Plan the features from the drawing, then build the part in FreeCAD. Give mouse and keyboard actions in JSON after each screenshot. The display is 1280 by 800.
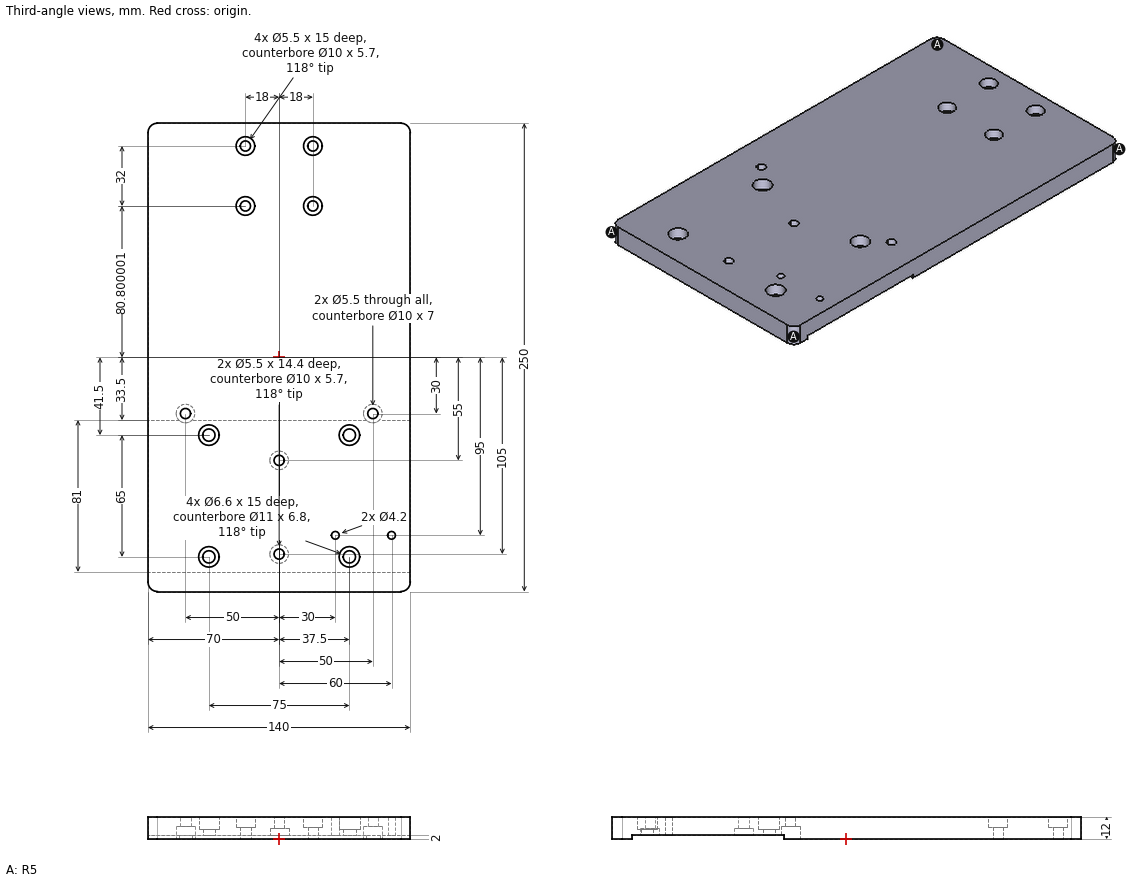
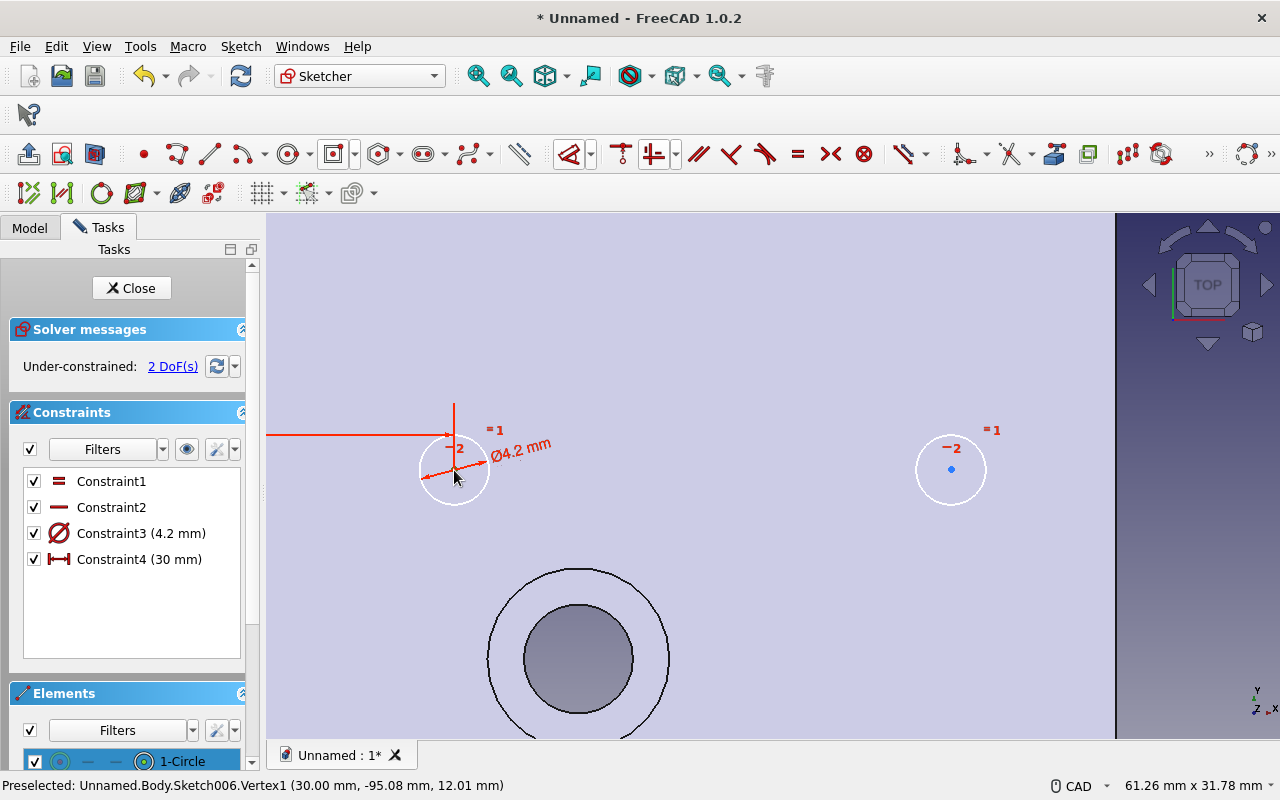
{"action": "left_click", "coordinate": [590, 154]}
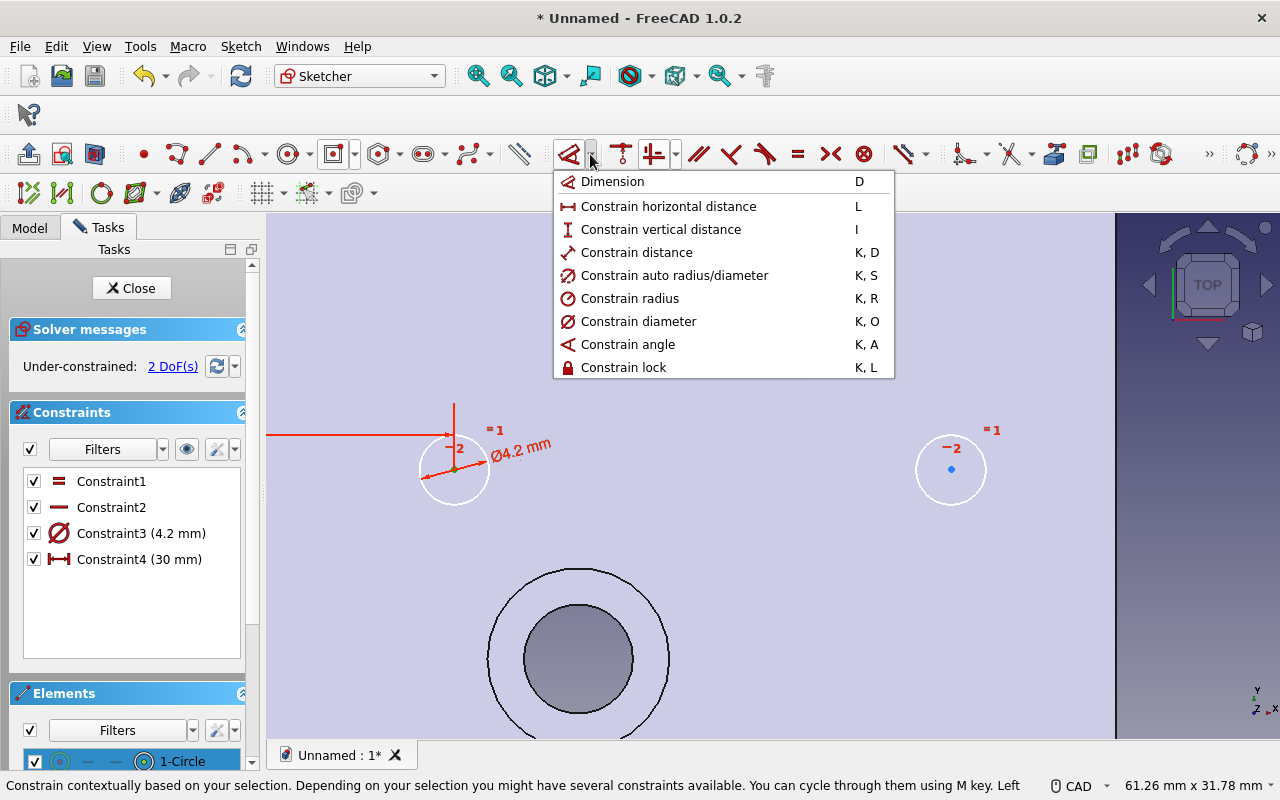
{"action": "left_click", "coordinate": [724, 230]}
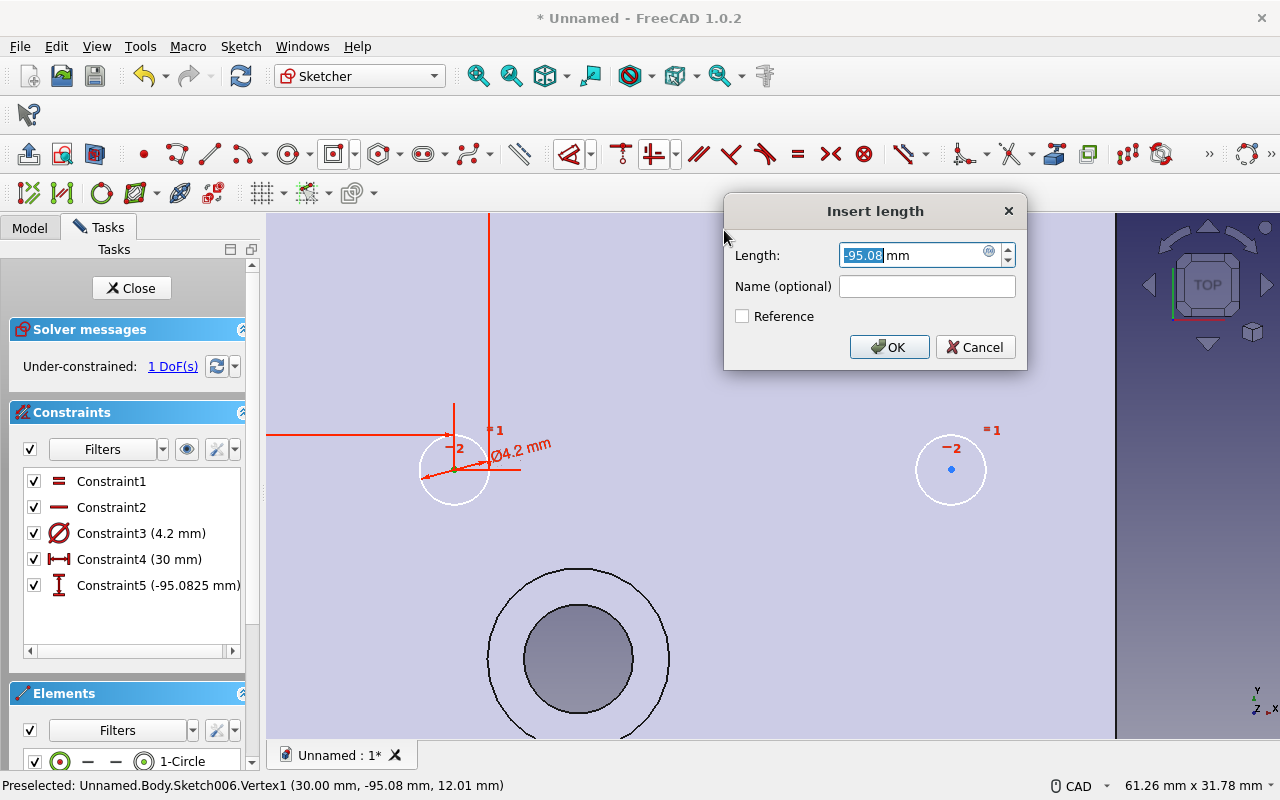
{"action": "type", "text": "-95"}
{"action": "key", "text": "Return"}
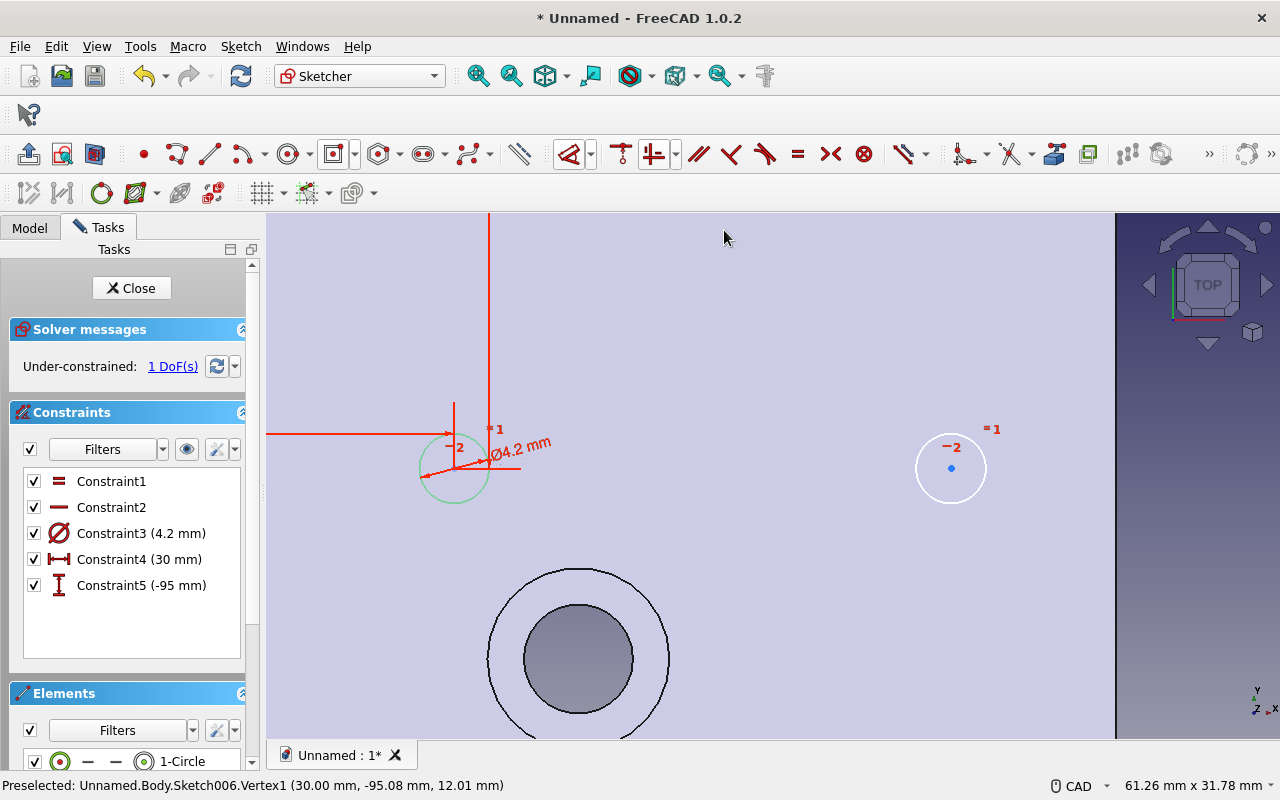
{"action": "left_click", "coordinate": [951, 469]}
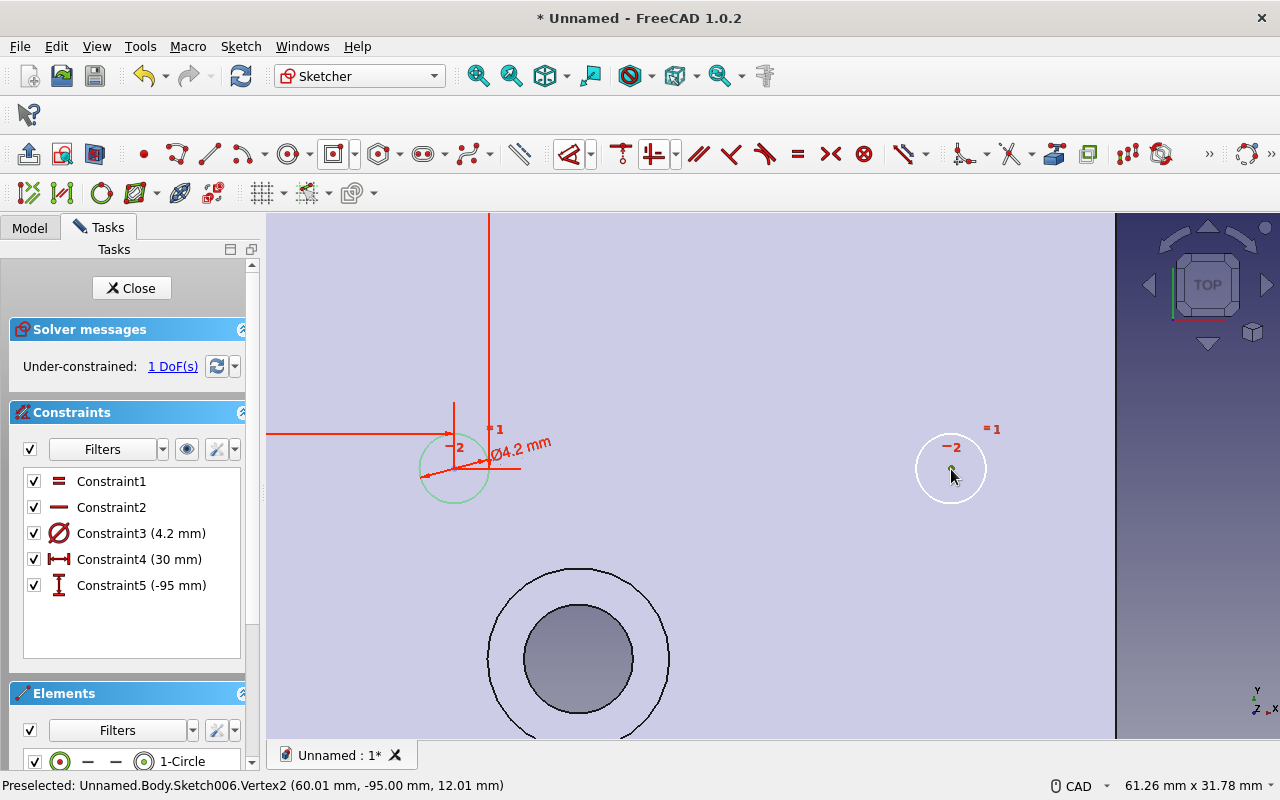
{"action": "key", "text": "l"}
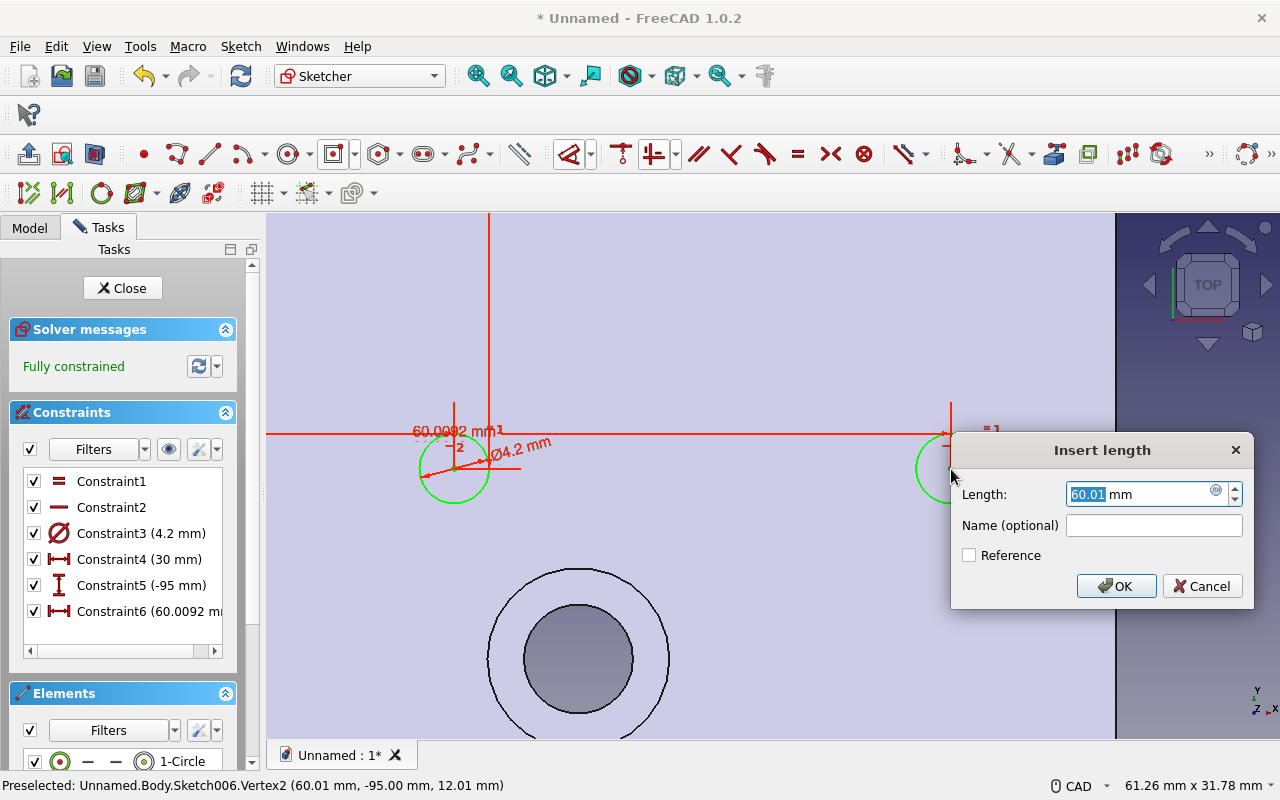
{"action": "type", "text": "60"}
{"action": "key", "text": "Return"}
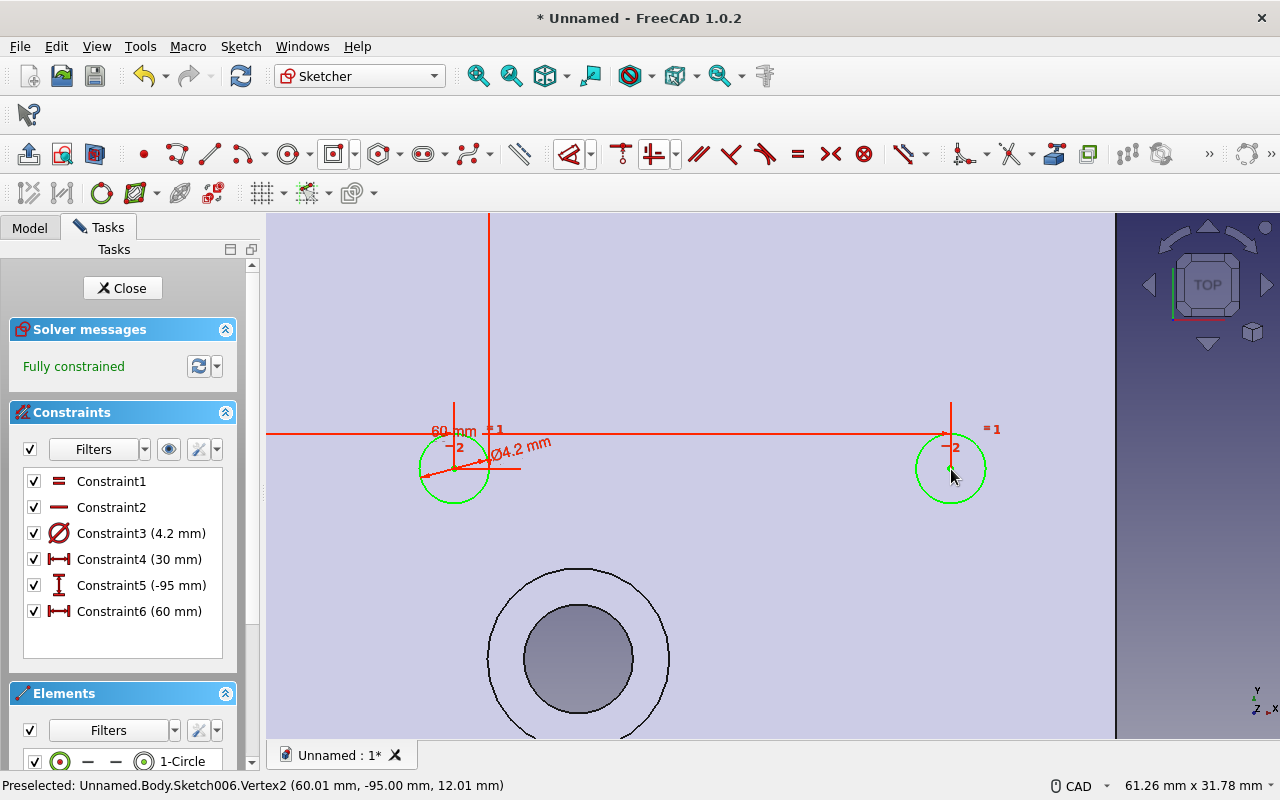
{"action": "left_click", "coordinate": [123, 288]}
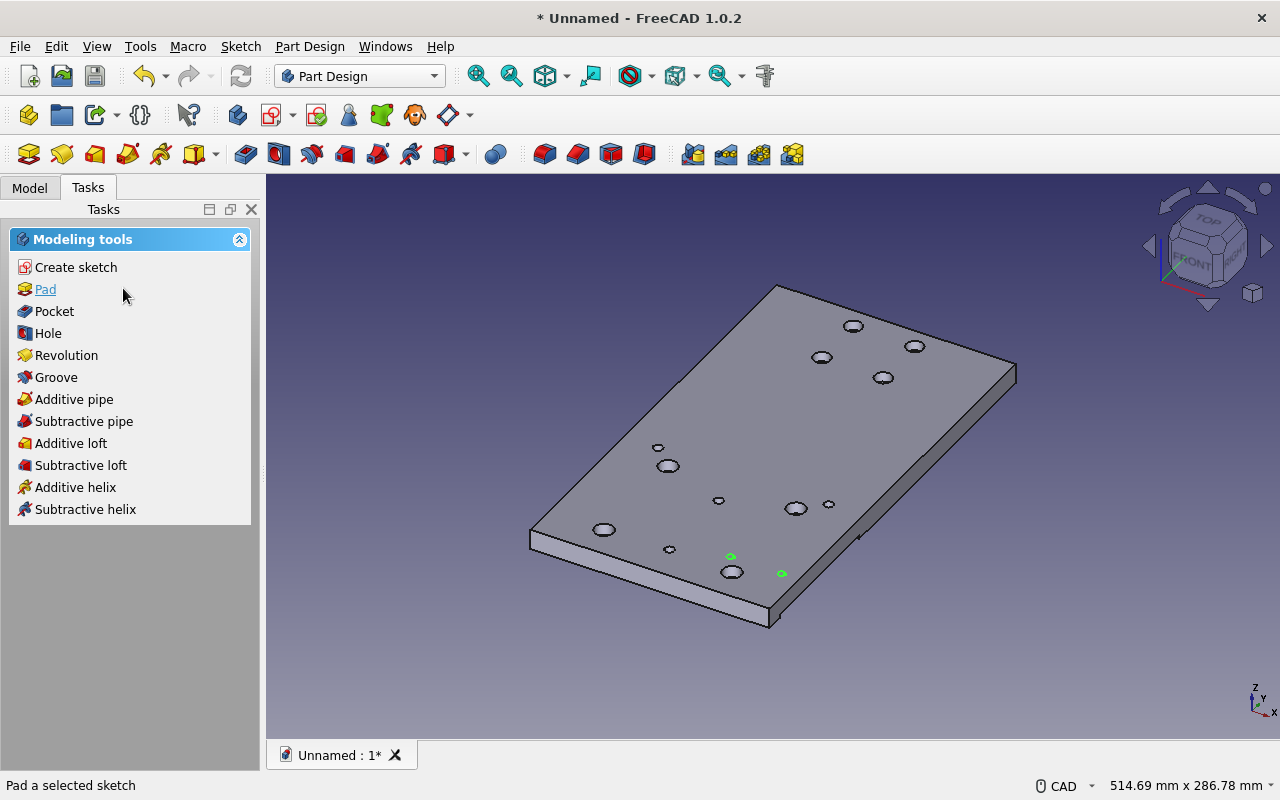
{"action": "left_click", "coordinate": [246, 154]}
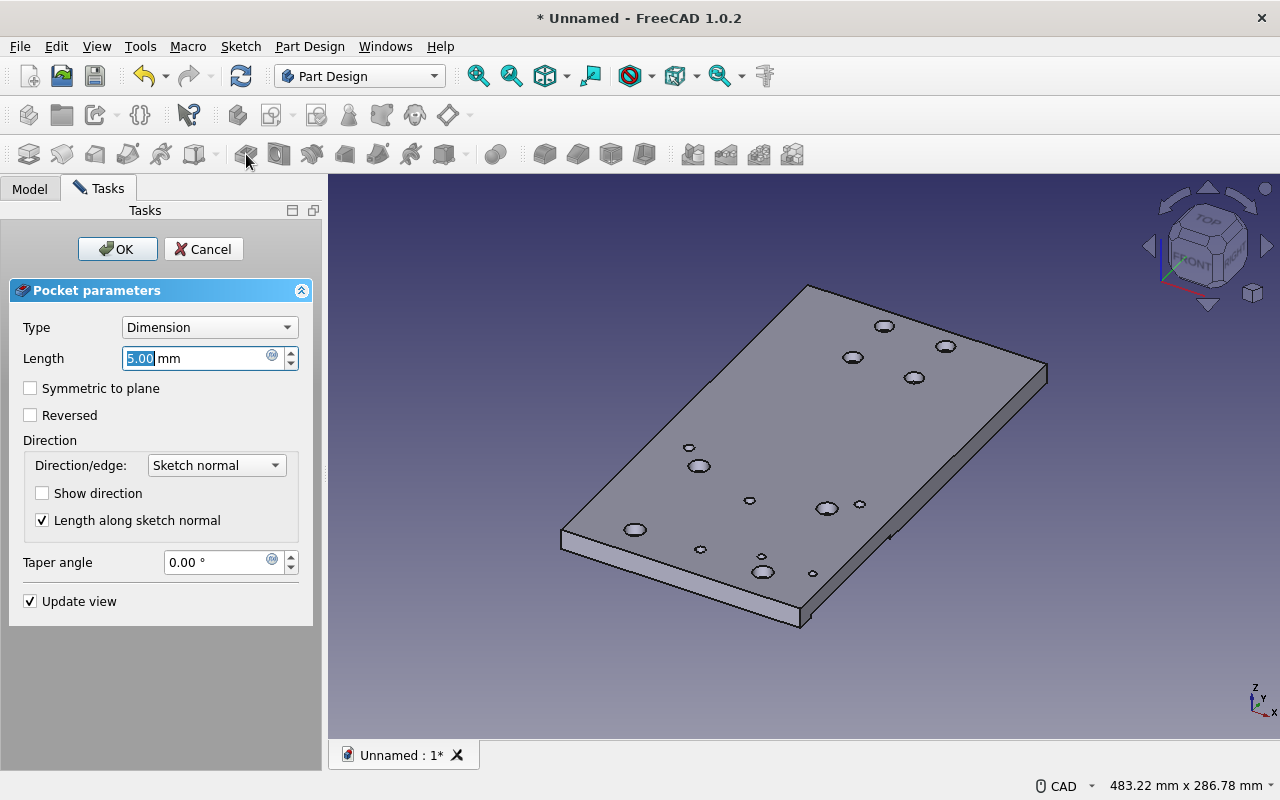
{"action": "left_click", "coordinate": [210, 328]}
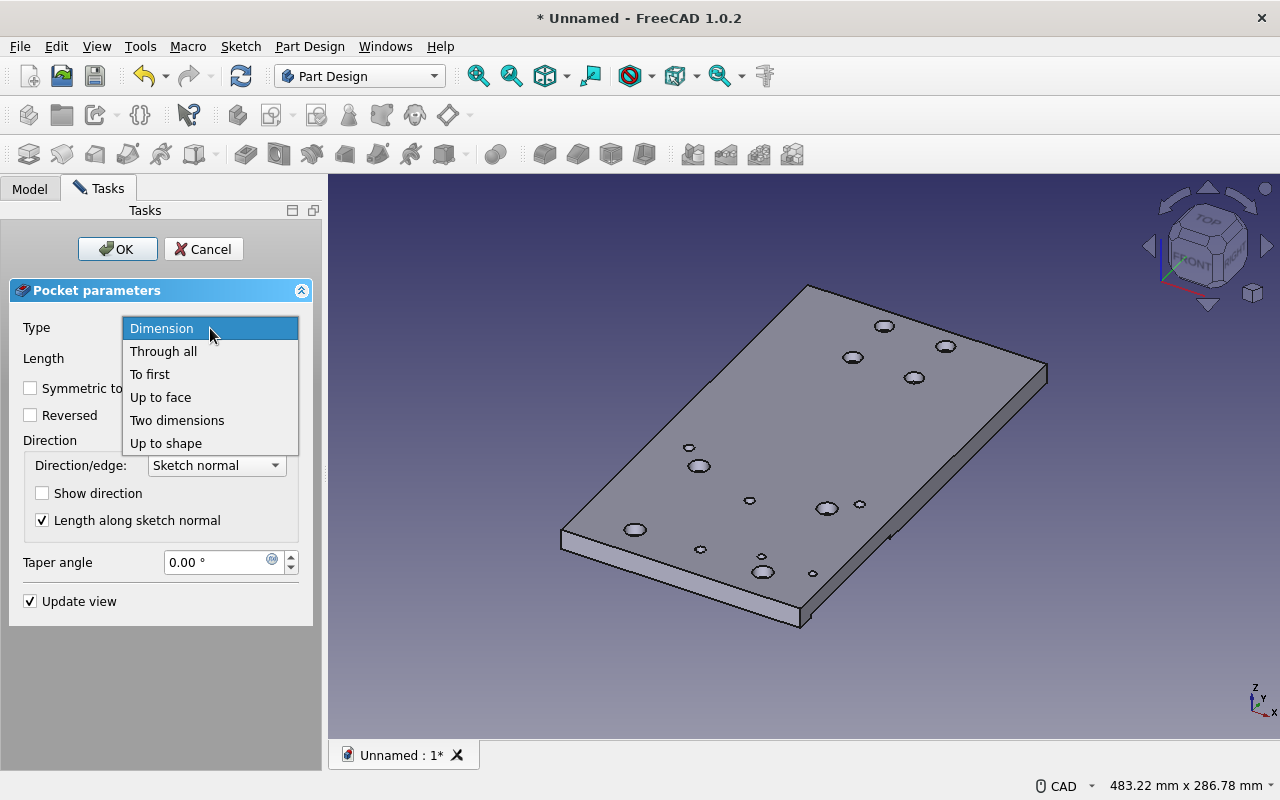
{"action": "left_click", "coordinate": [208, 352]}